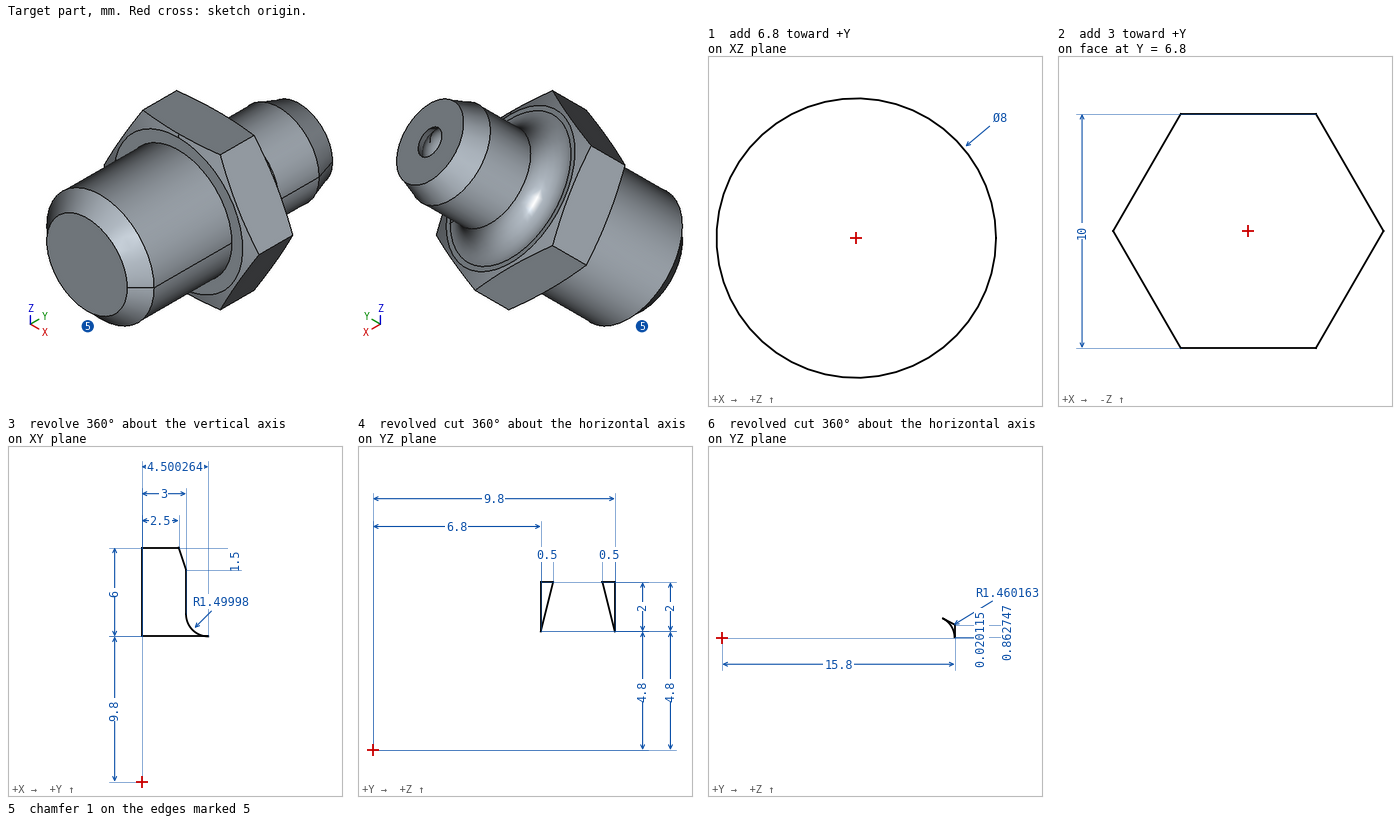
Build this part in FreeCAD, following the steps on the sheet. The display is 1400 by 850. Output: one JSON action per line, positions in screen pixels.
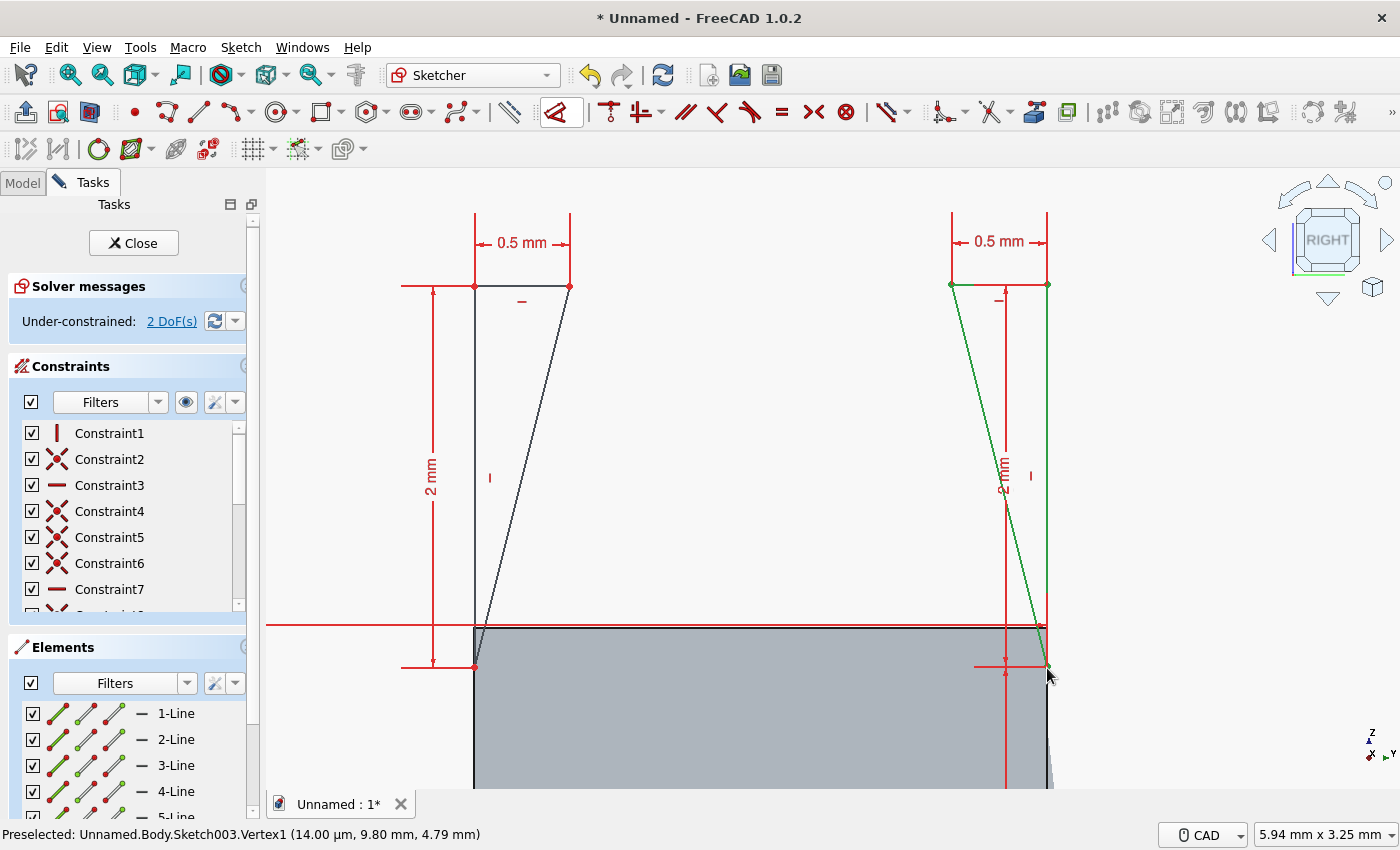
{"action": "left_click", "coordinate": [475, 668]}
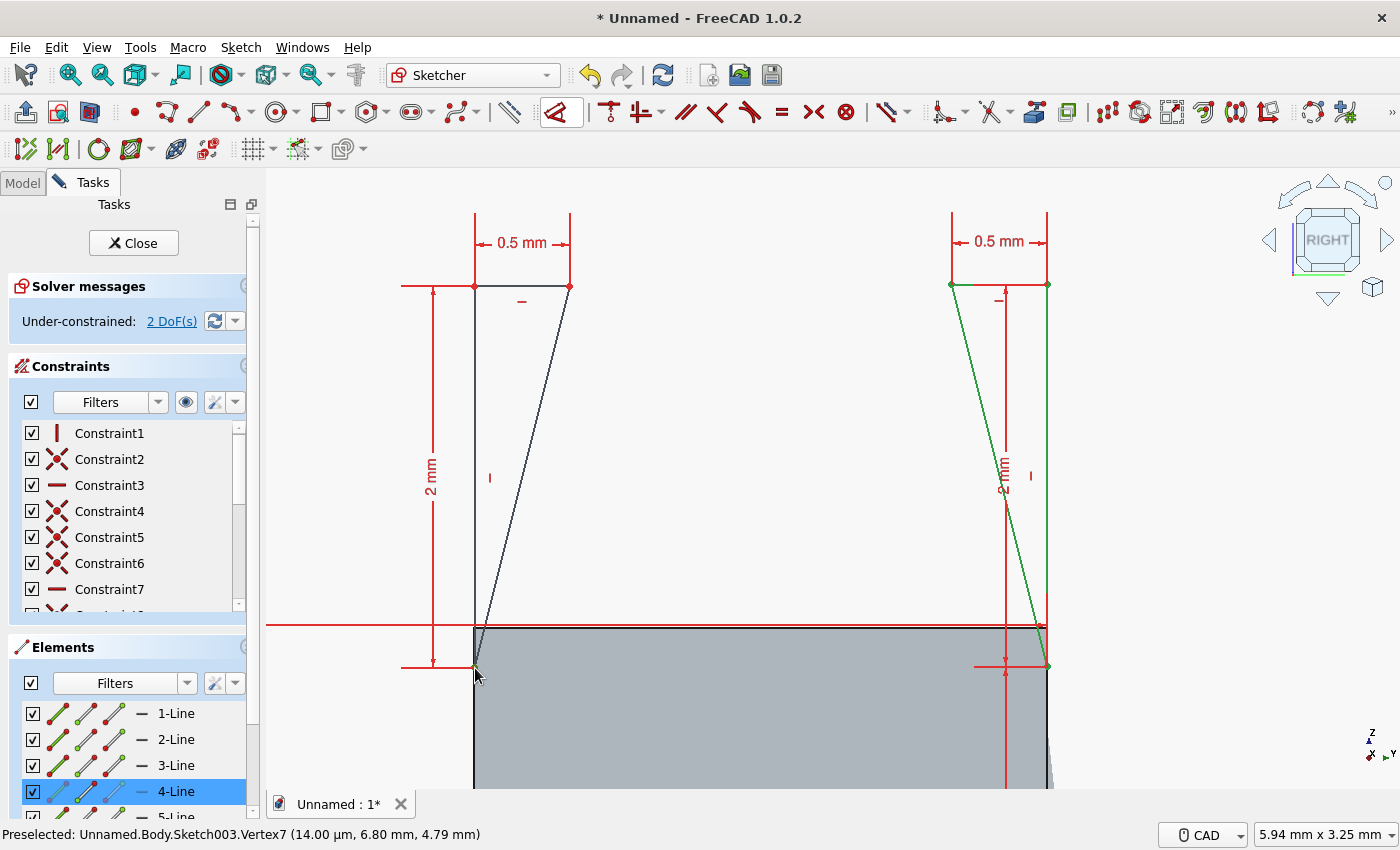
{"action": "left_click", "coordinate": [578, 112]}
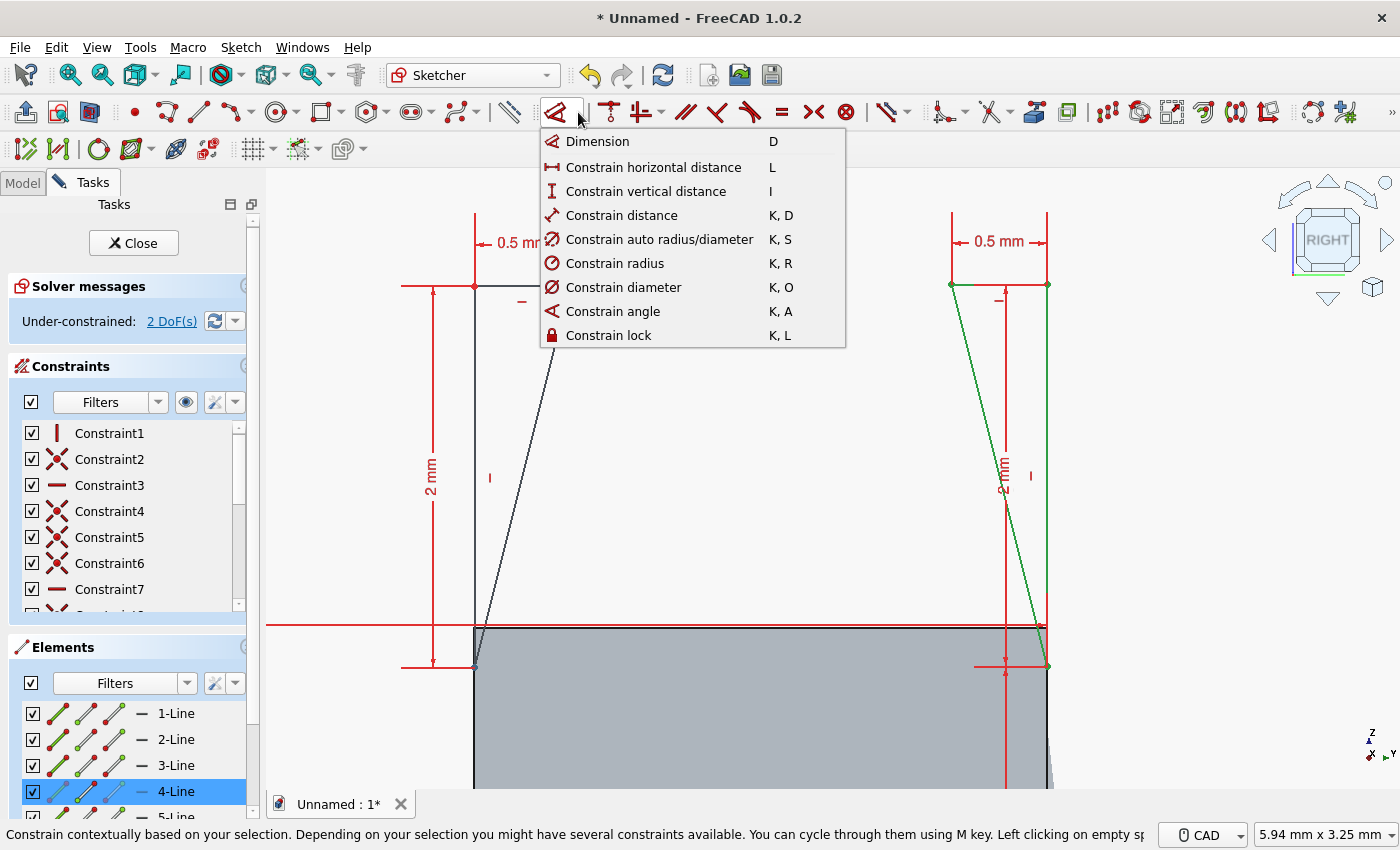
{"action": "left_click", "coordinate": [693, 167]}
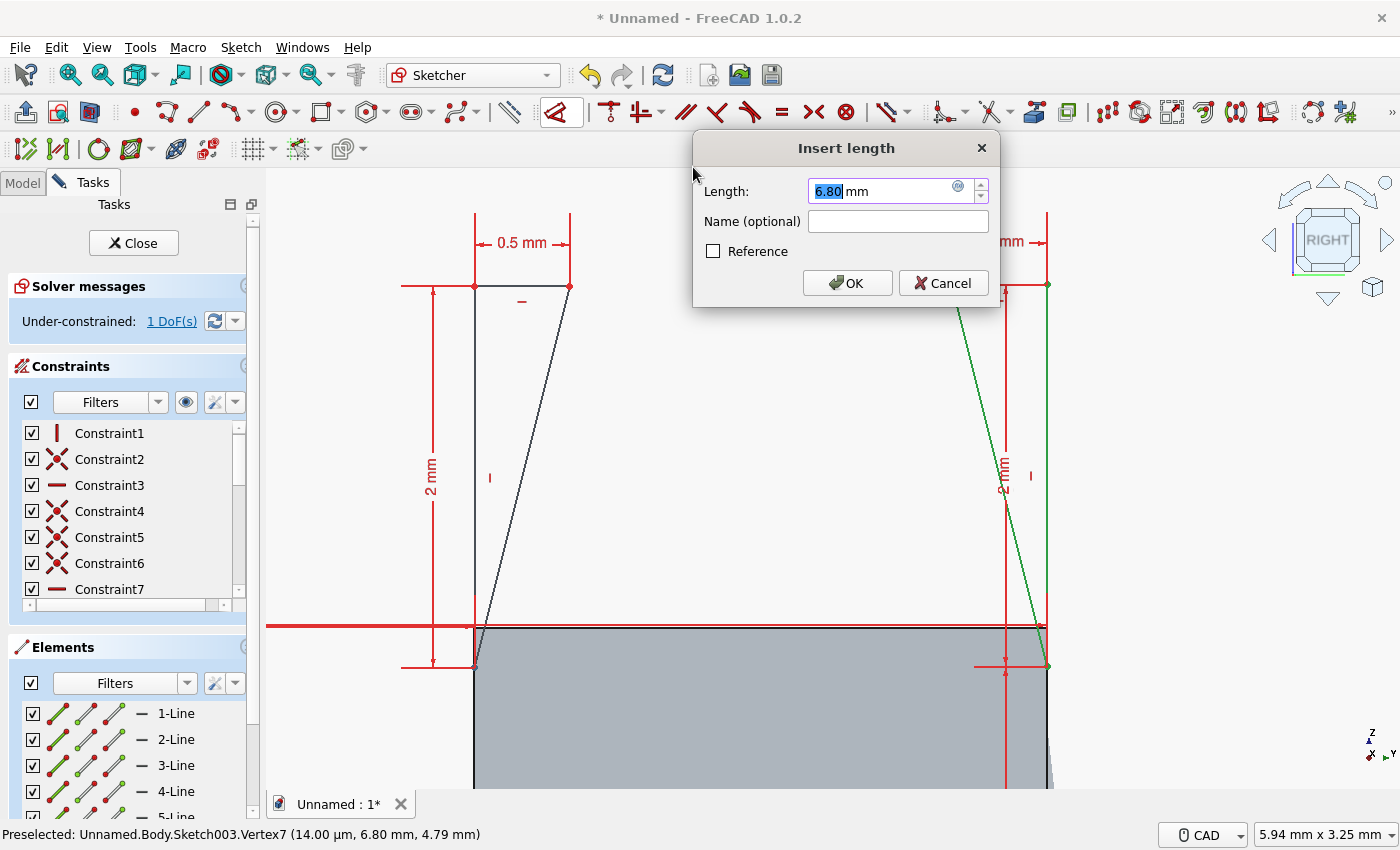
{"action": "type", "text": "6.8"}
{"action": "key", "text": "Return"}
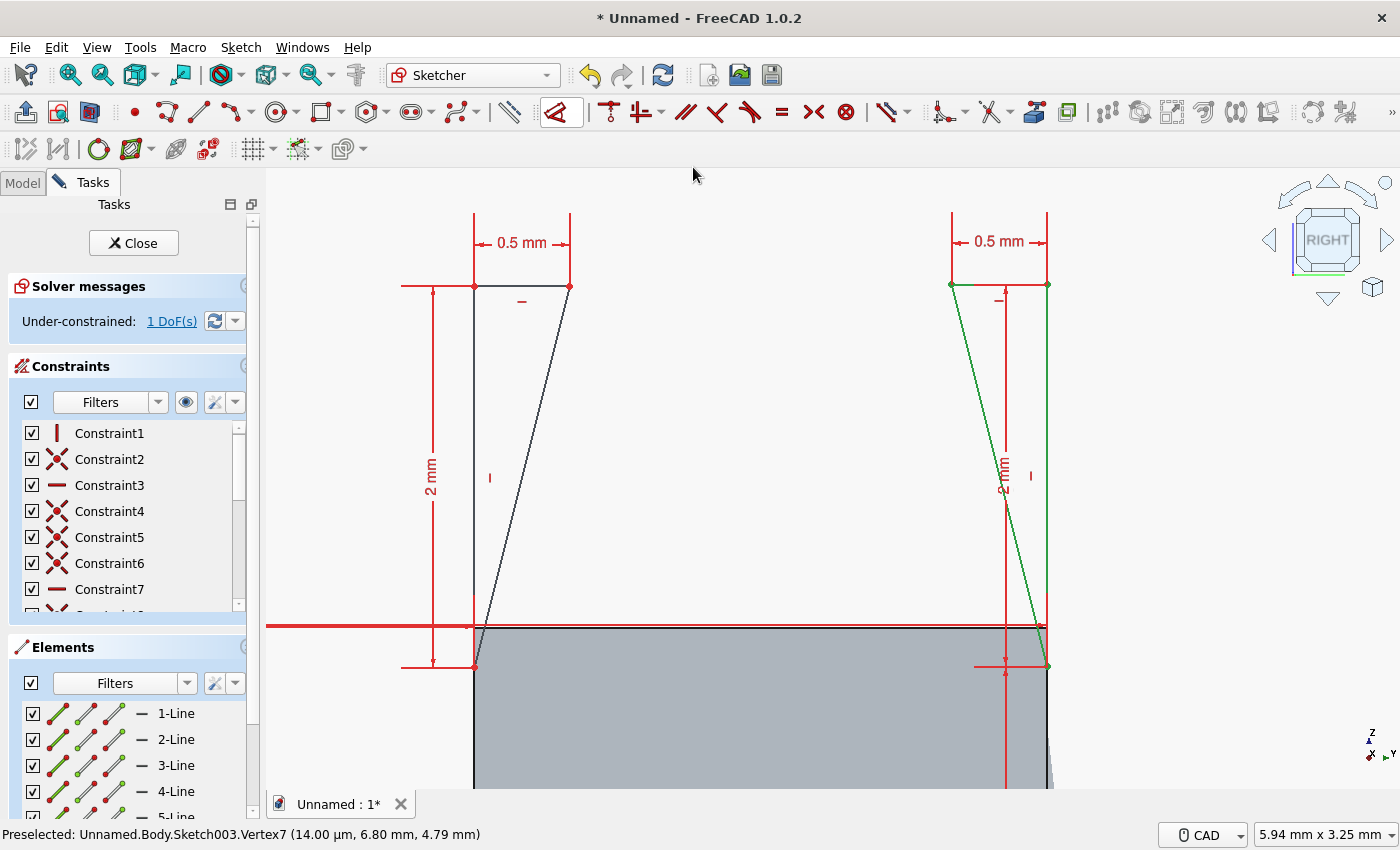
{"action": "left_click", "coordinate": [474, 668]}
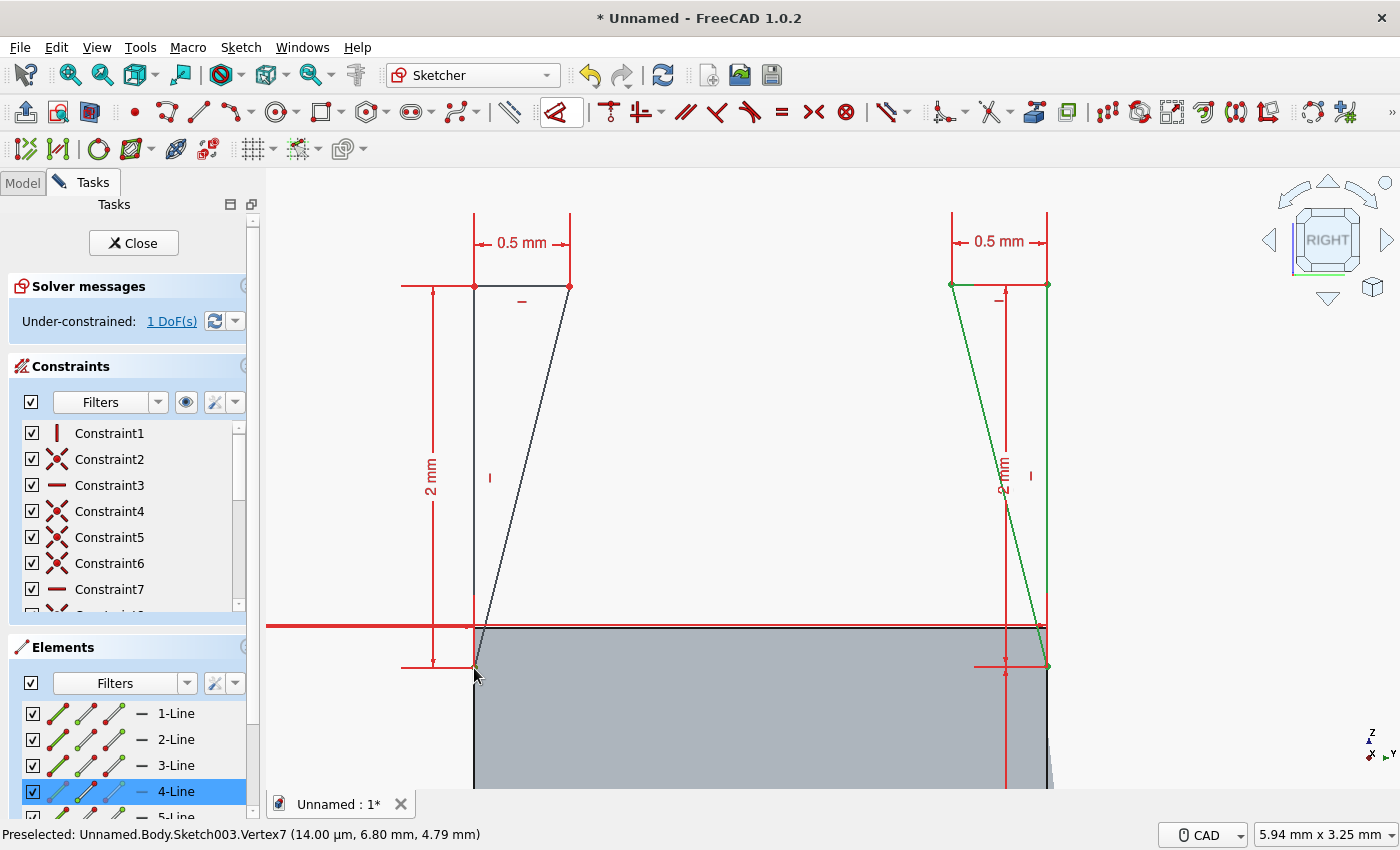
{"action": "key", "text": "i"}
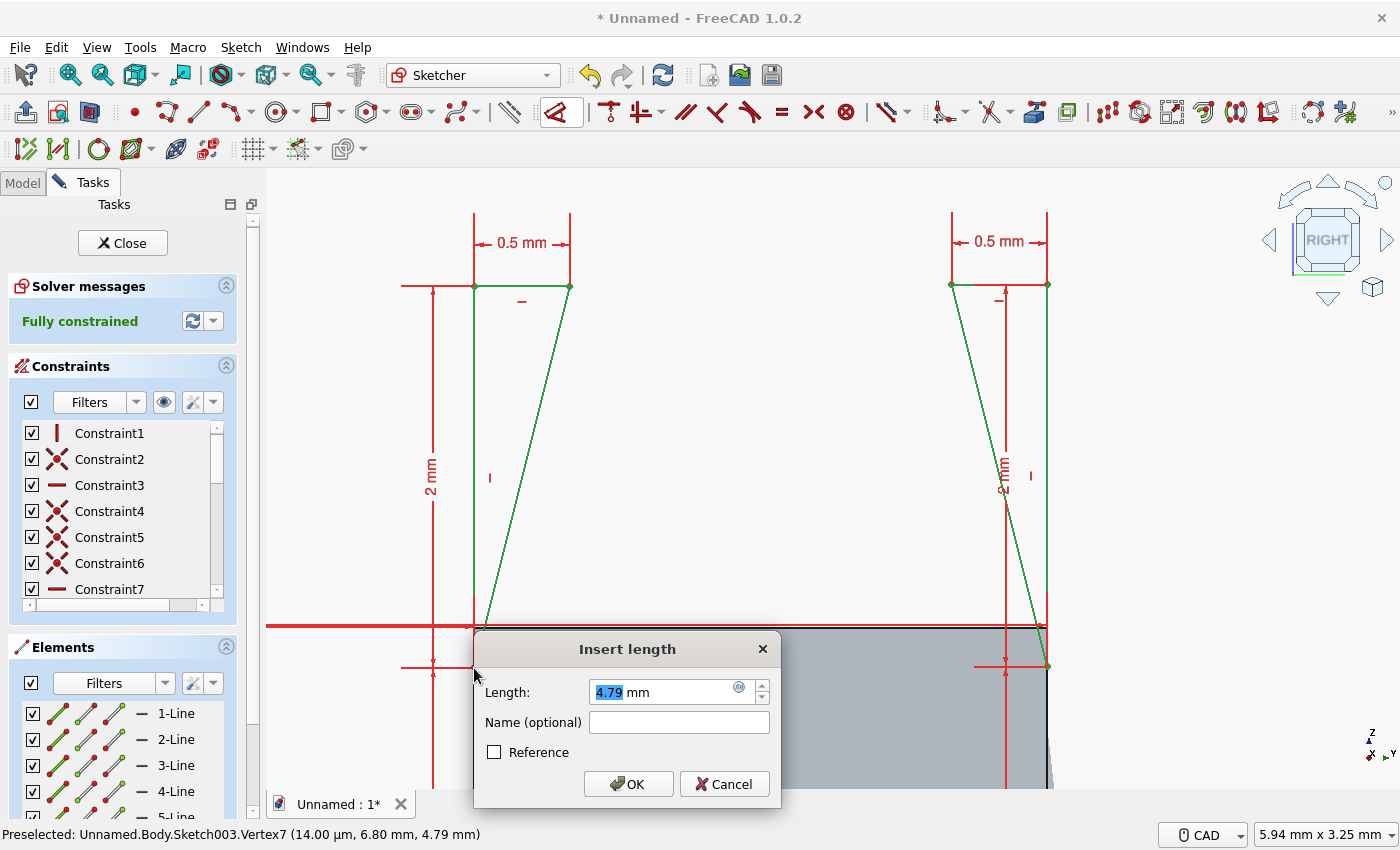
{"action": "type", "text": "4.8"}
{"action": "key", "text": "Return"}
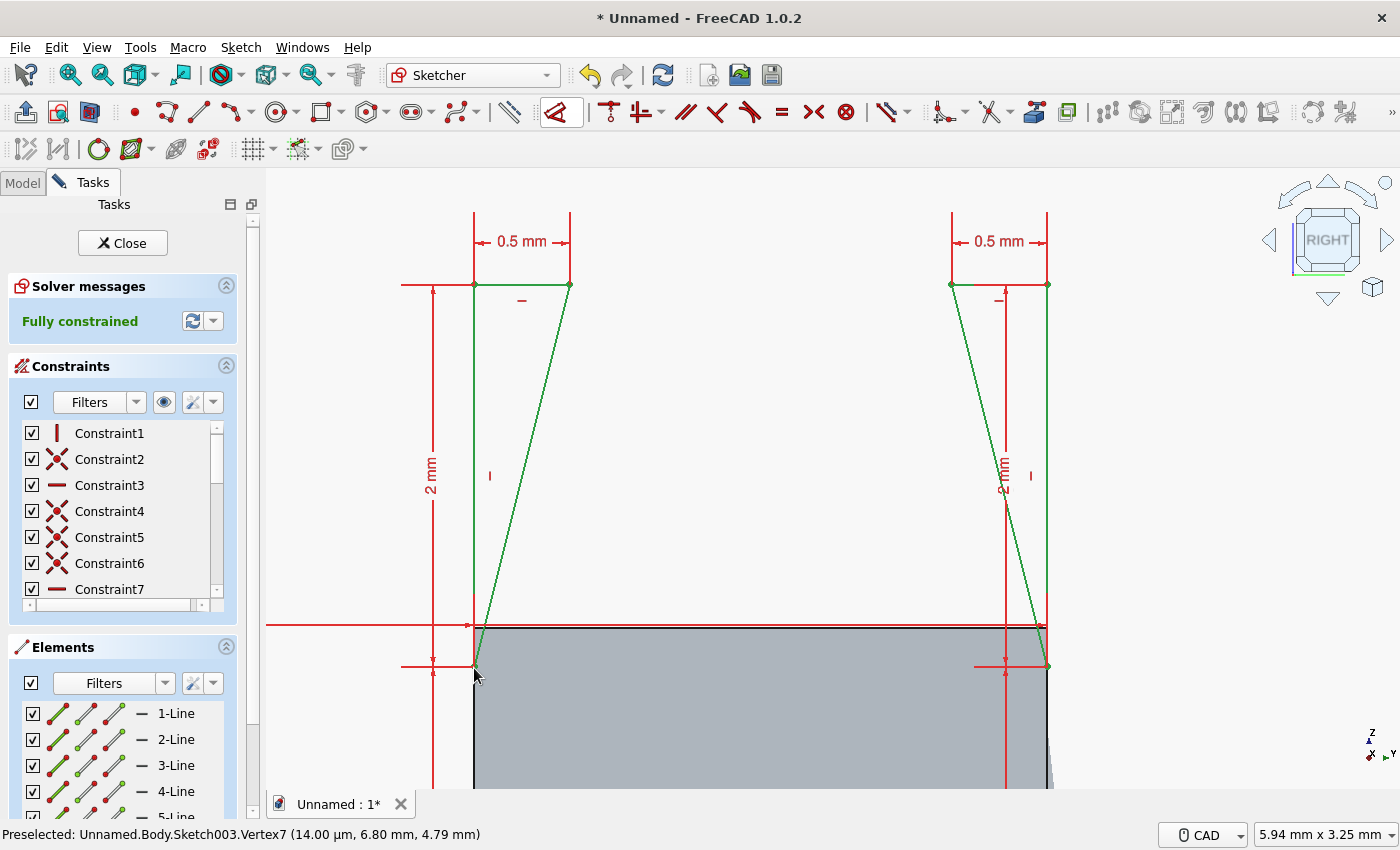
{"action": "left_click", "coordinate": [123, 243]}